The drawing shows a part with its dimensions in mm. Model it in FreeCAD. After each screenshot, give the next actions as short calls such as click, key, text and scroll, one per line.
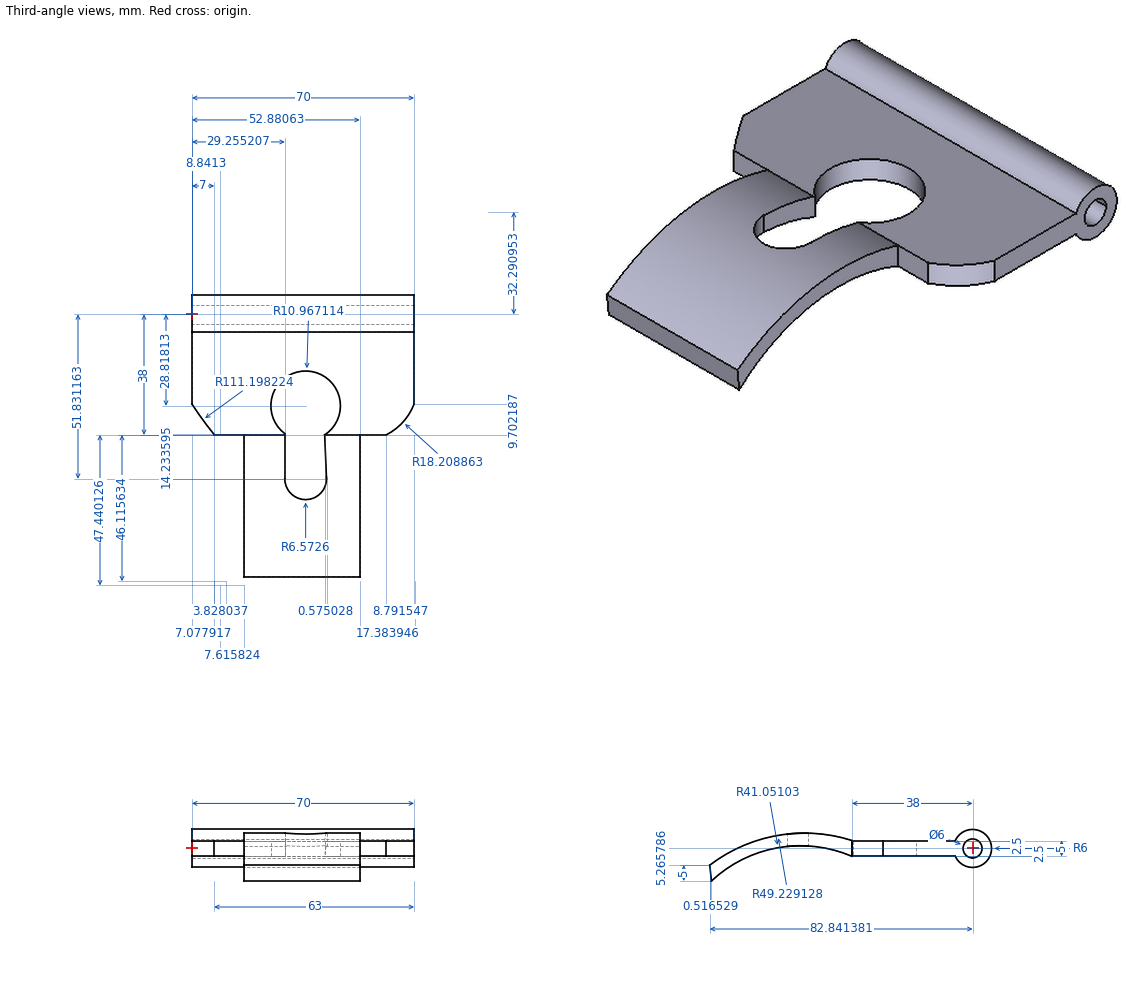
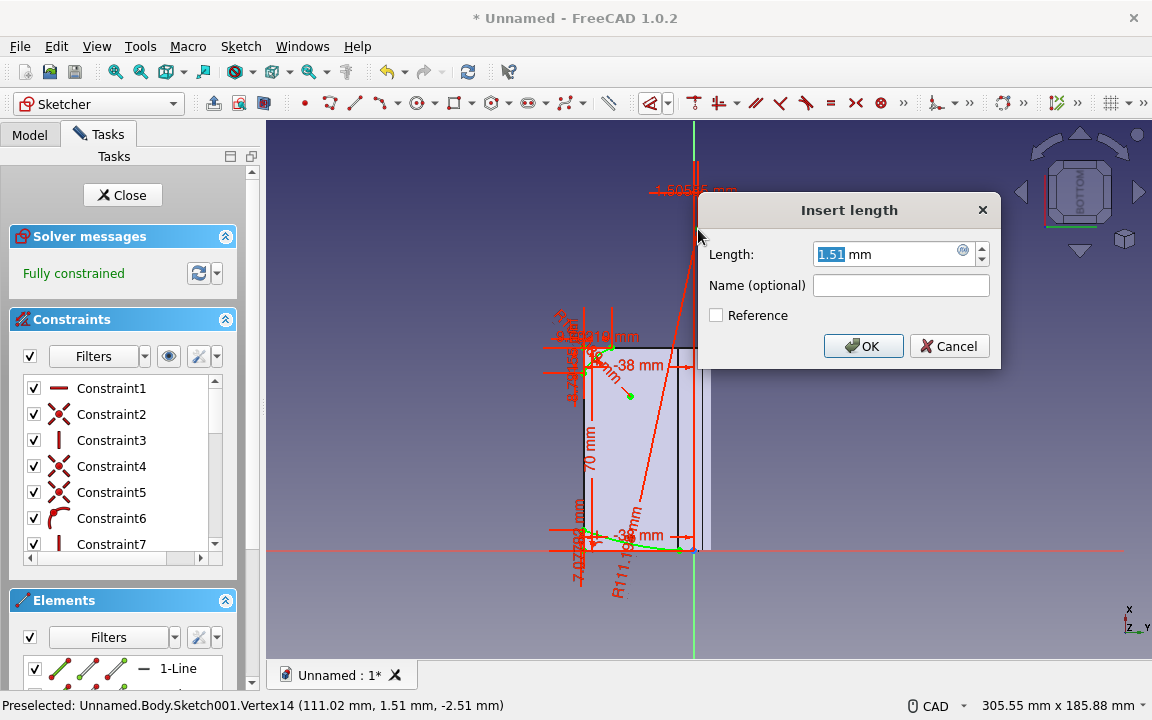
text(32.290953)
key(Return)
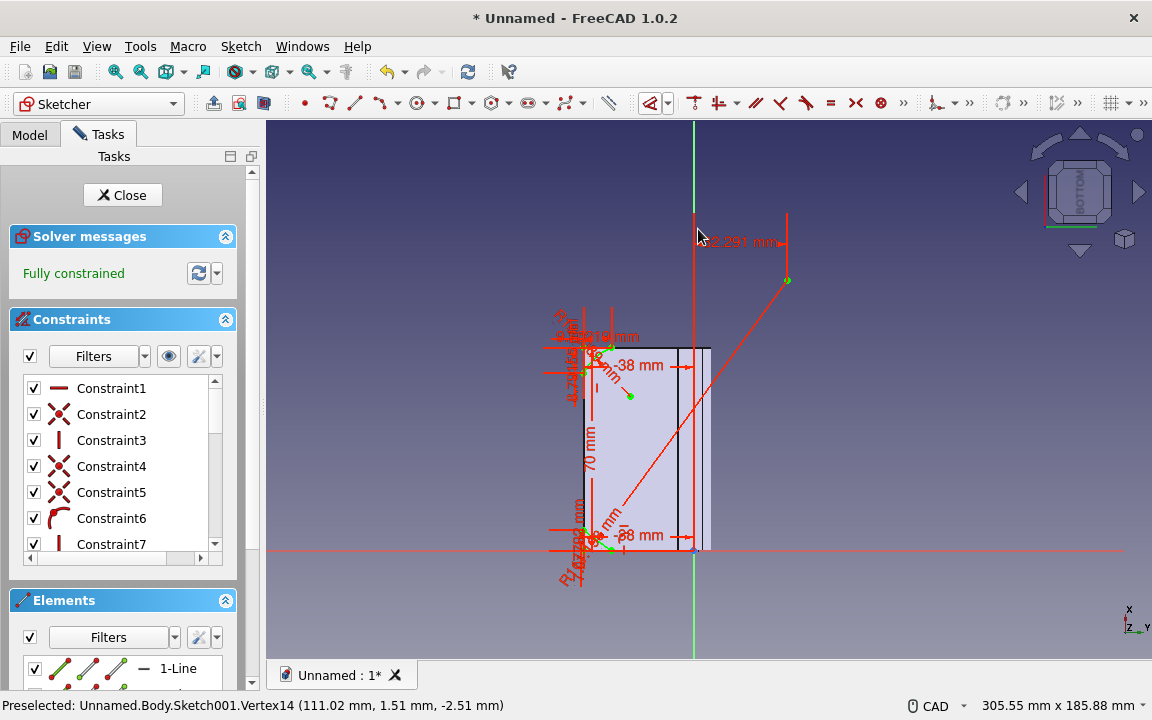
click(123, 195)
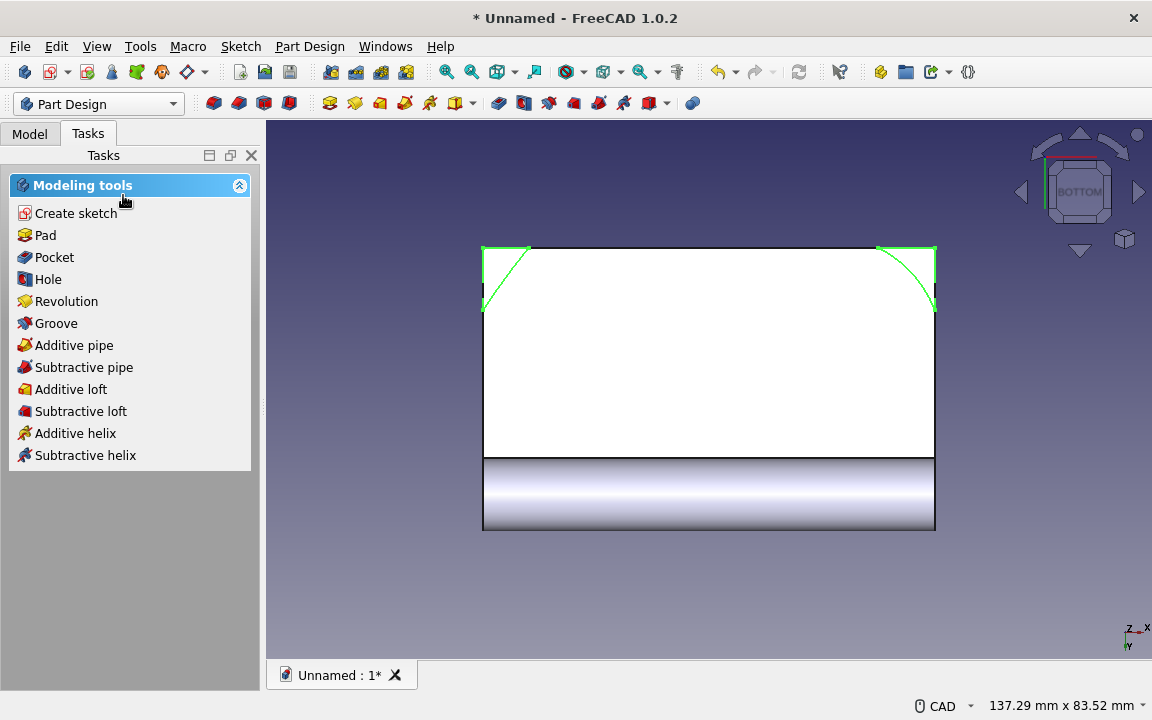
click(499, 104)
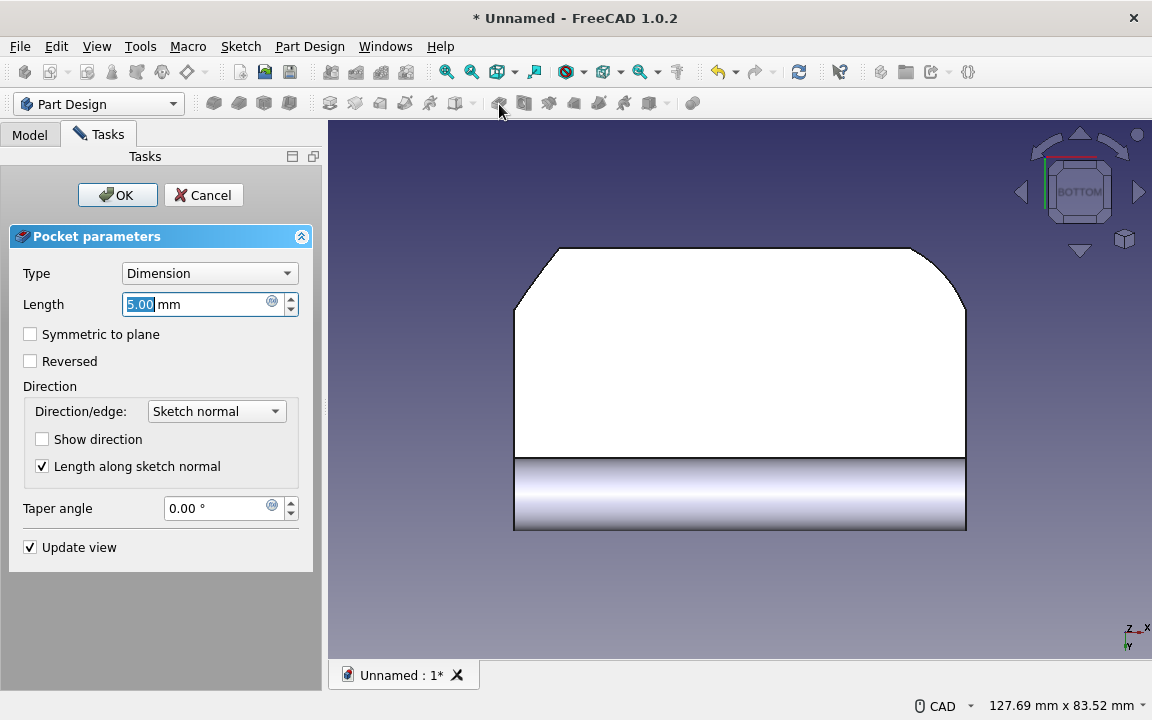
text(70)
key(Tab)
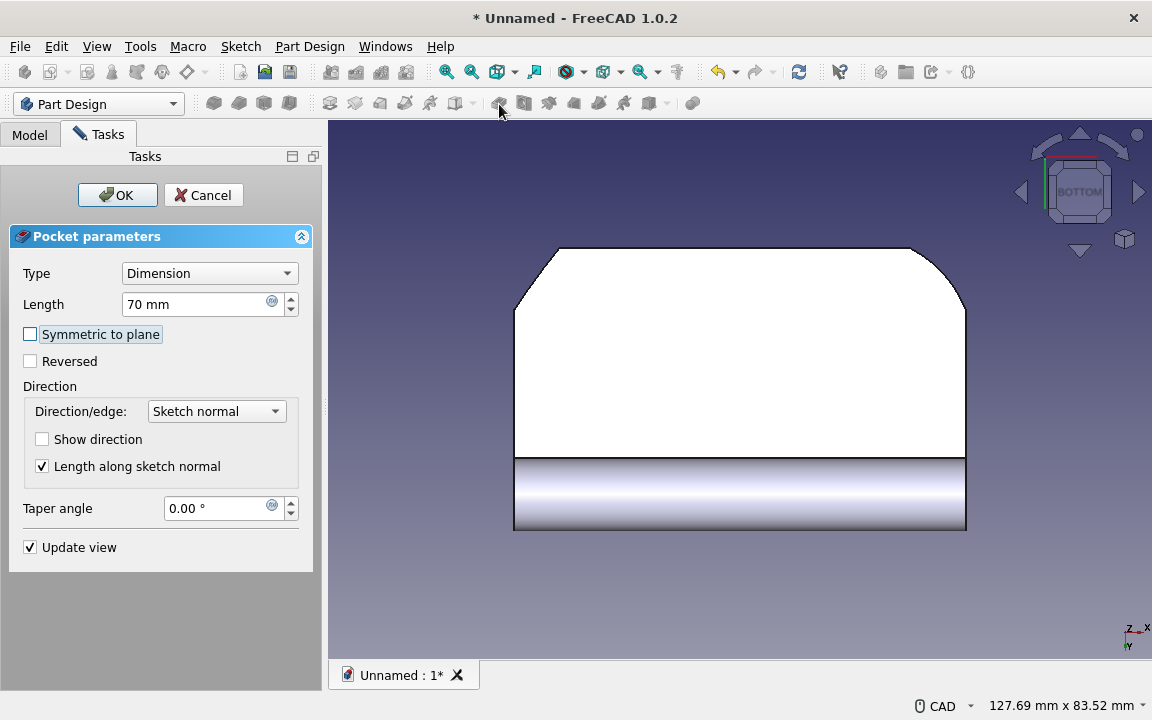
click(118, 195)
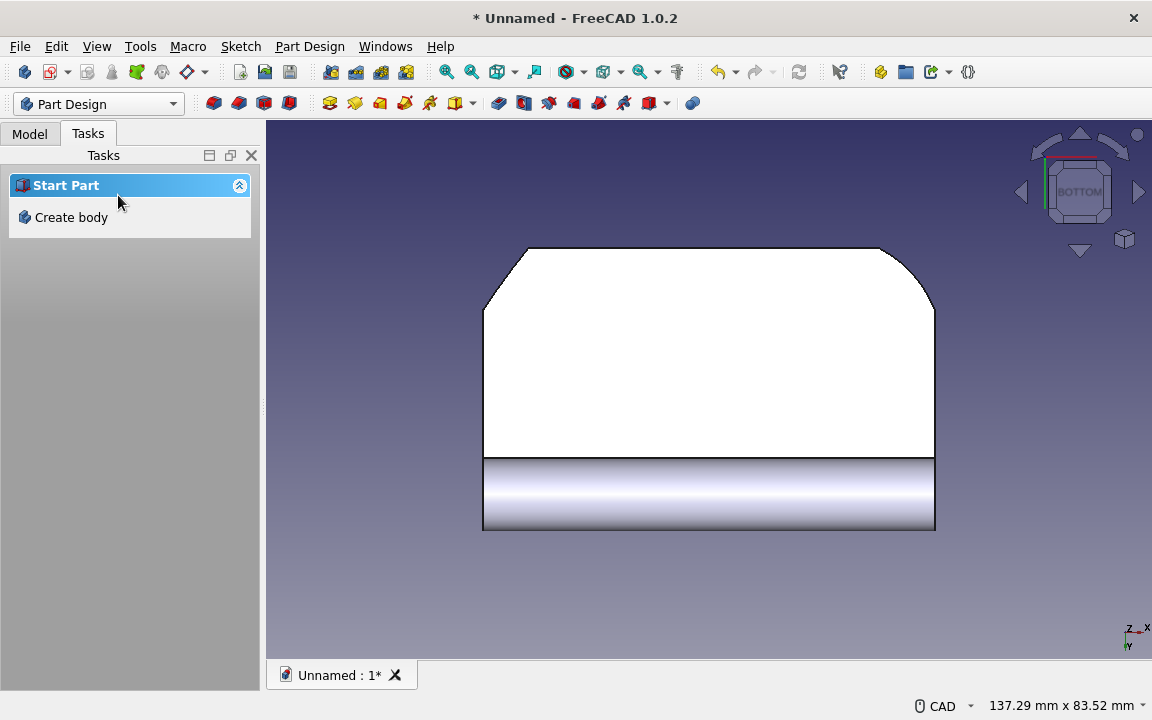
key(0)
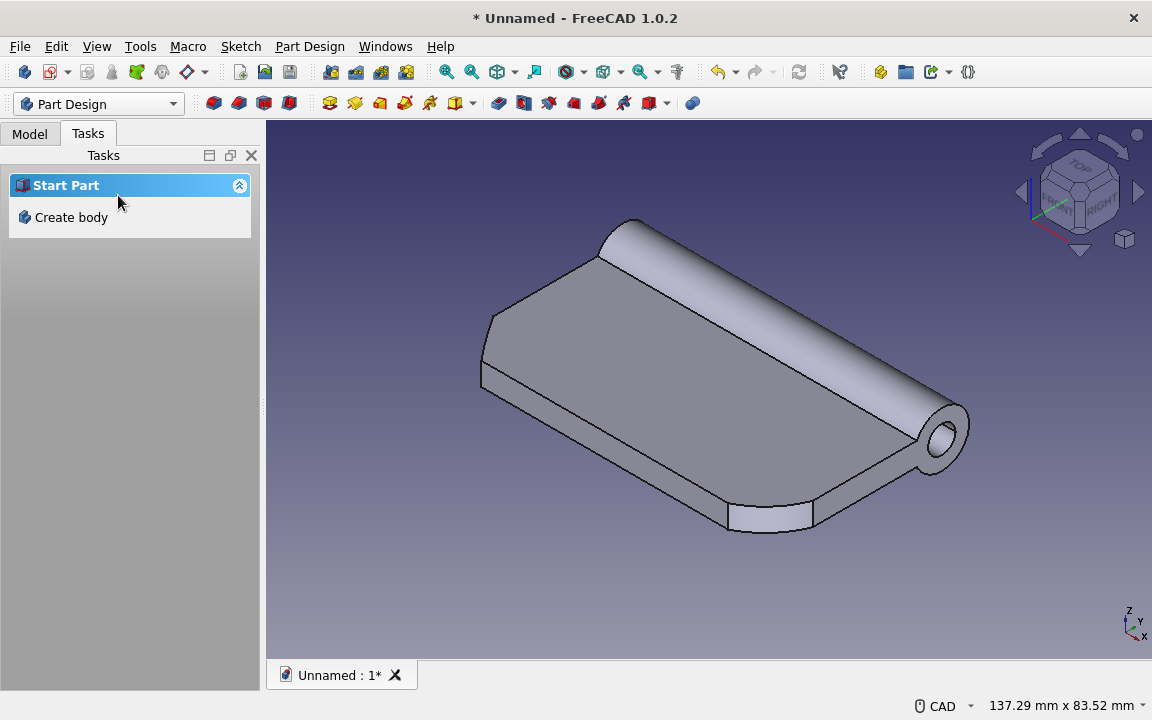
click(913, 455)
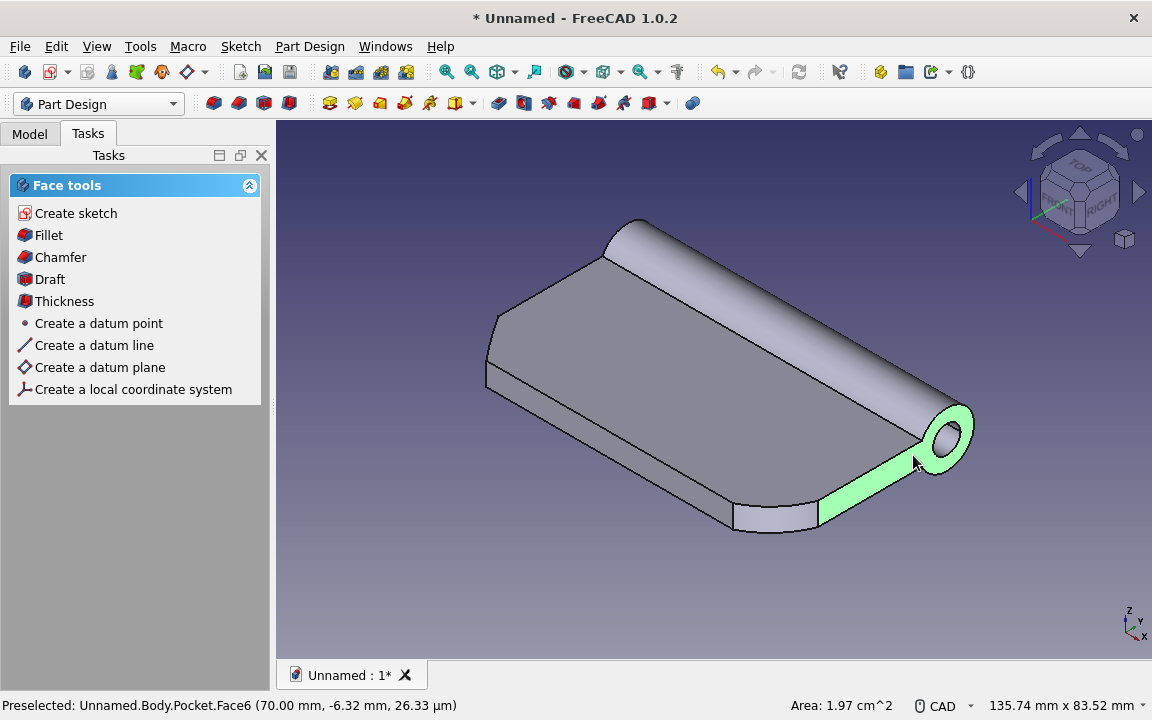
click(50, 72)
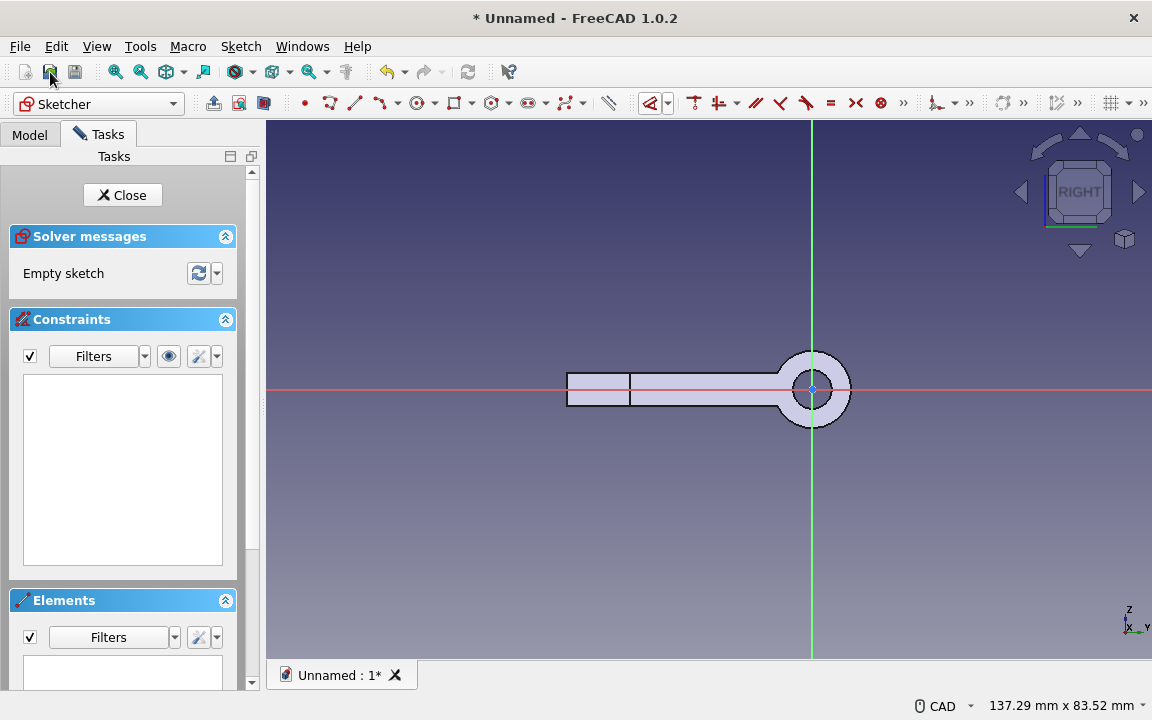
scroll(987, 300, down, 1)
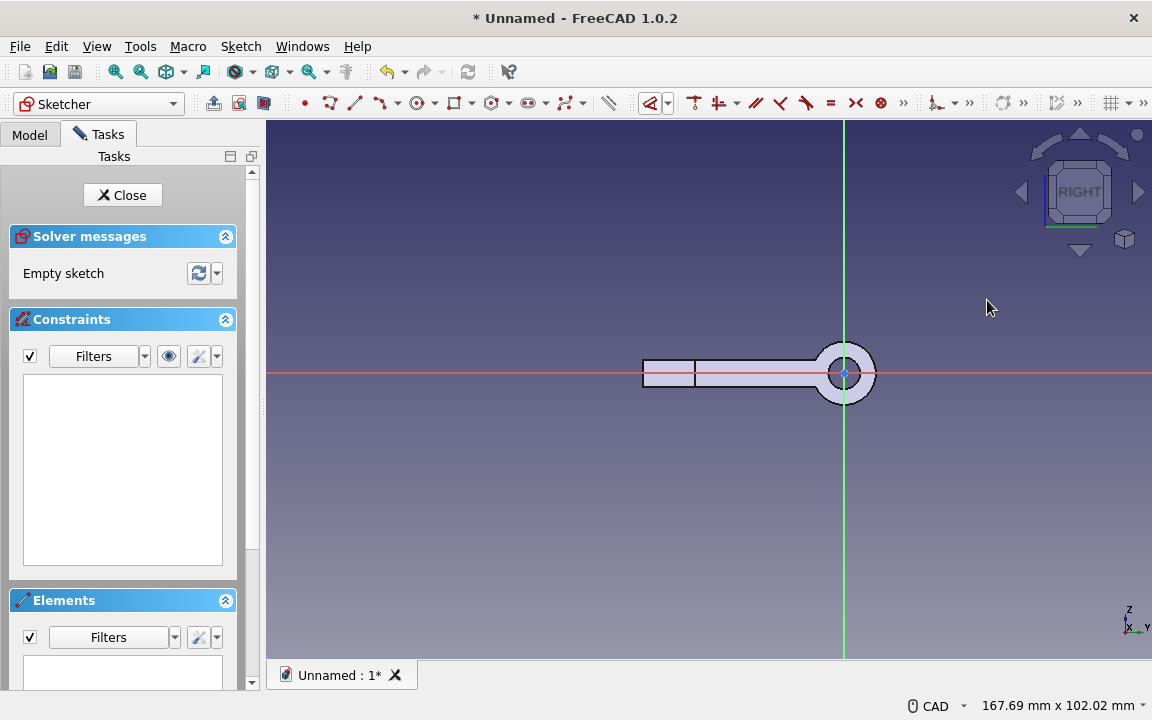
click(355, 104)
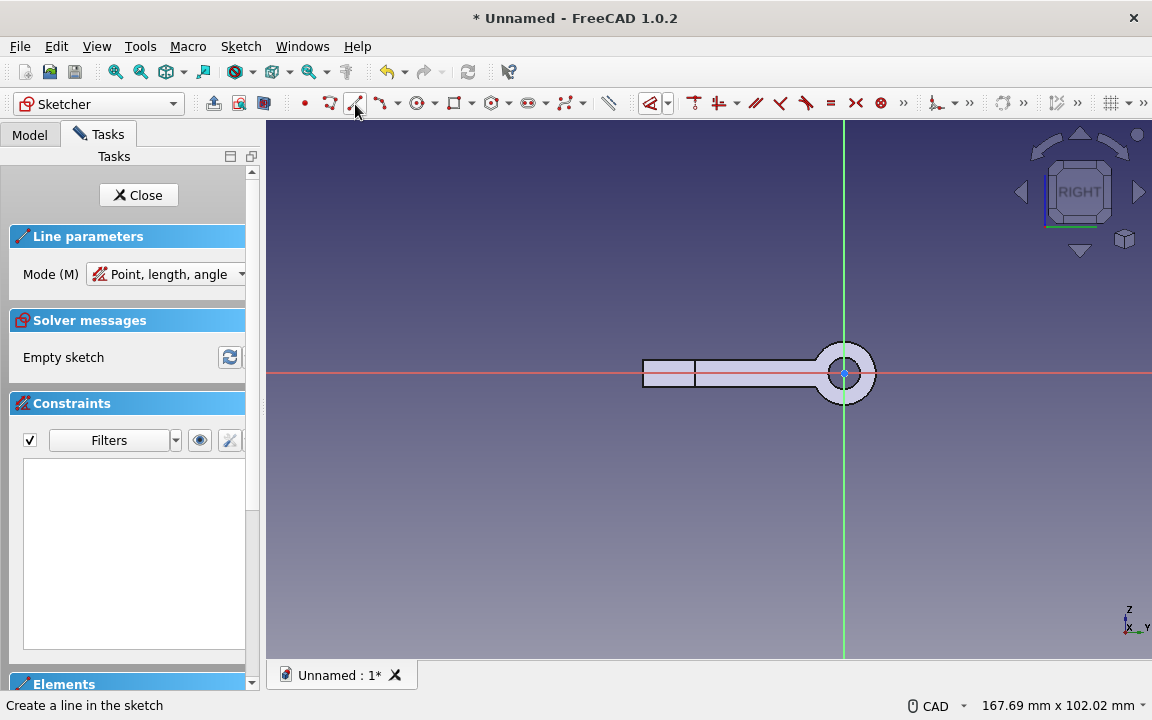
click(406, 401)
click(409, 428)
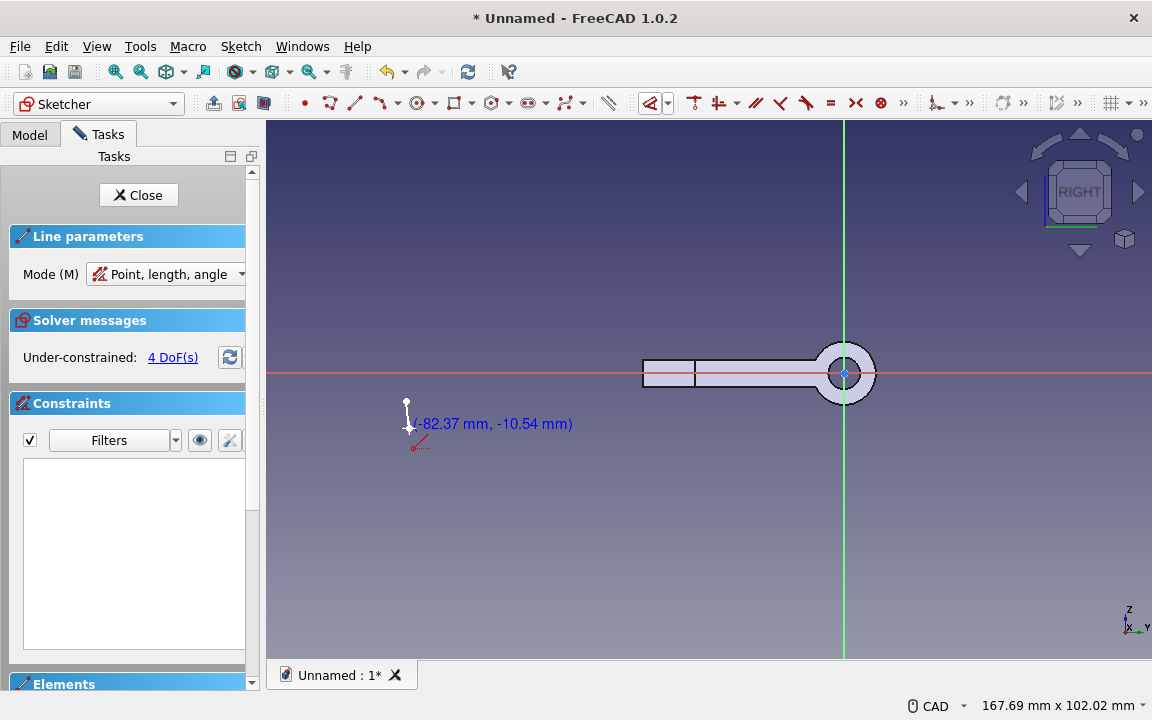
click(643, 387)
click(643, 360)